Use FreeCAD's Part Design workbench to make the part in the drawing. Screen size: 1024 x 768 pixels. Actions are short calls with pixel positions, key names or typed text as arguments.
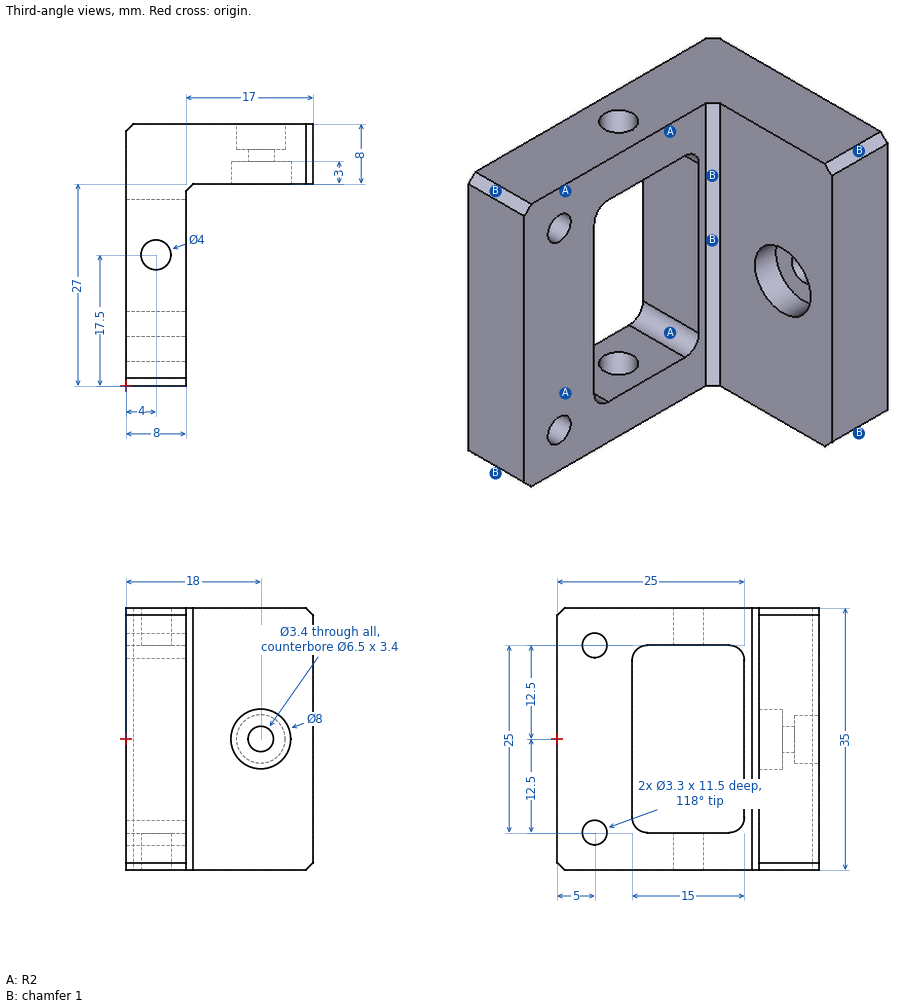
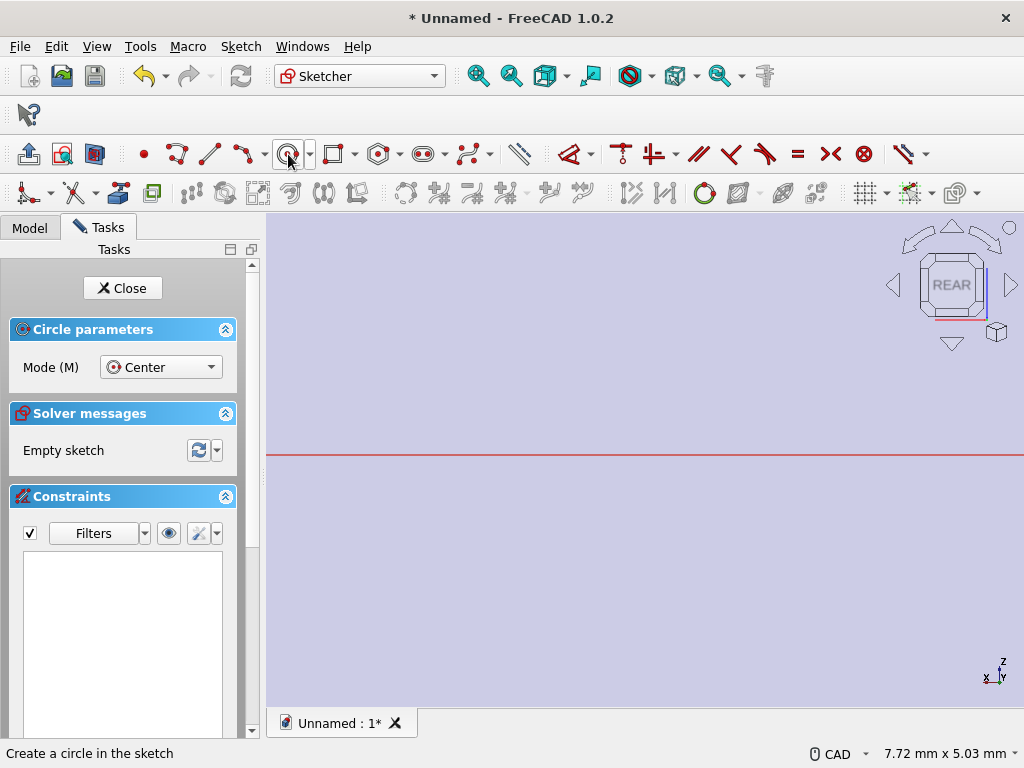
click(572, 455)
move(690, 337)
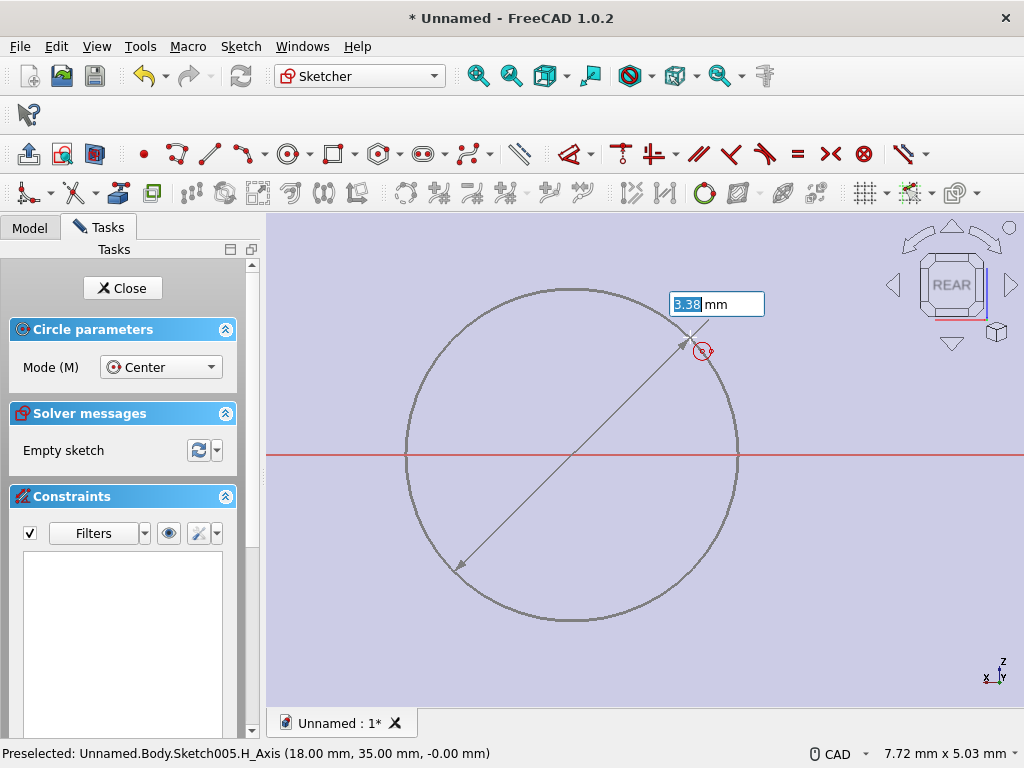
text(3.4)
key(Return)
key(Escape)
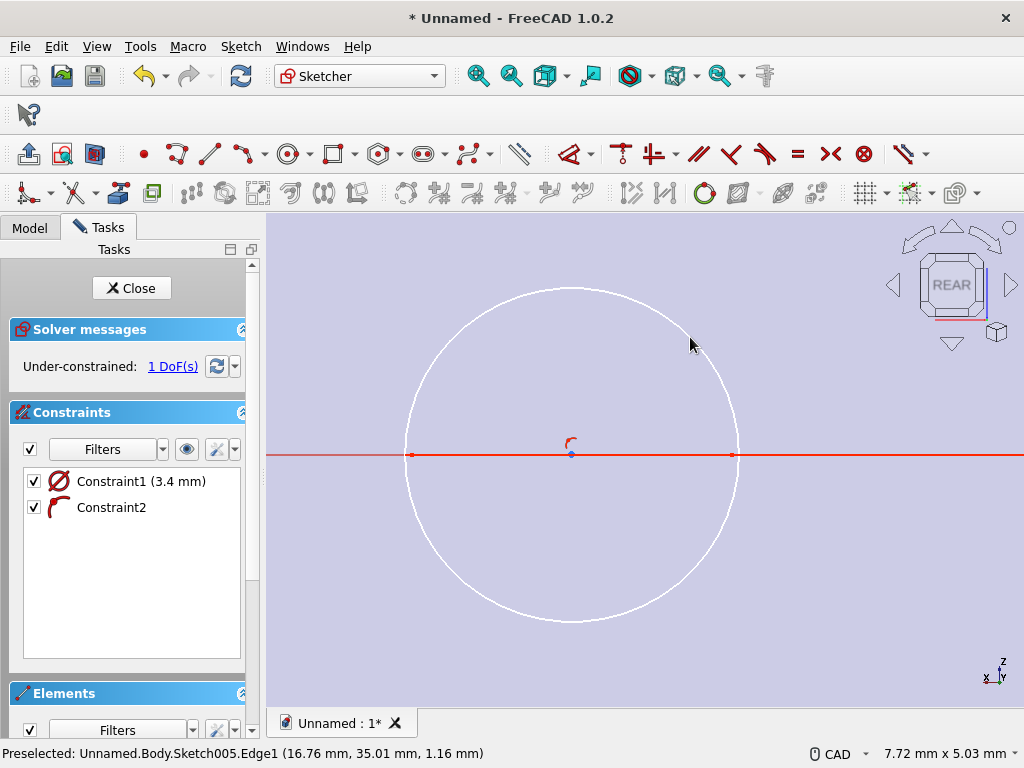
key(d)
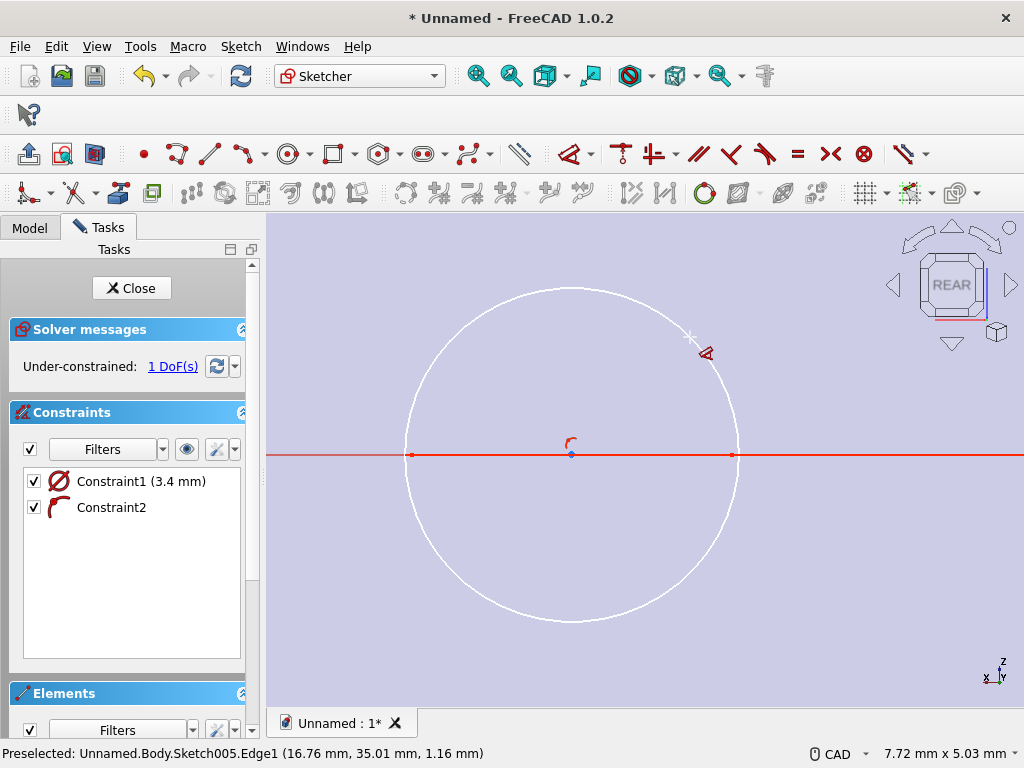
click(572, 455)
click(716, 489)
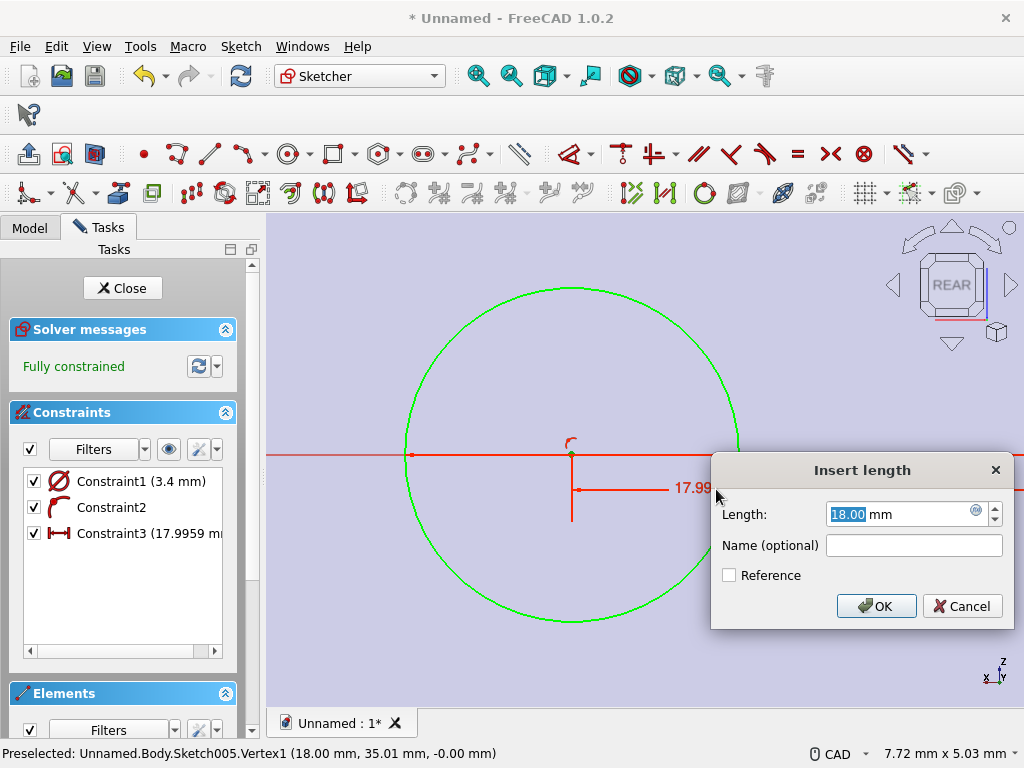
text(18)
key(Return)
key(Escape)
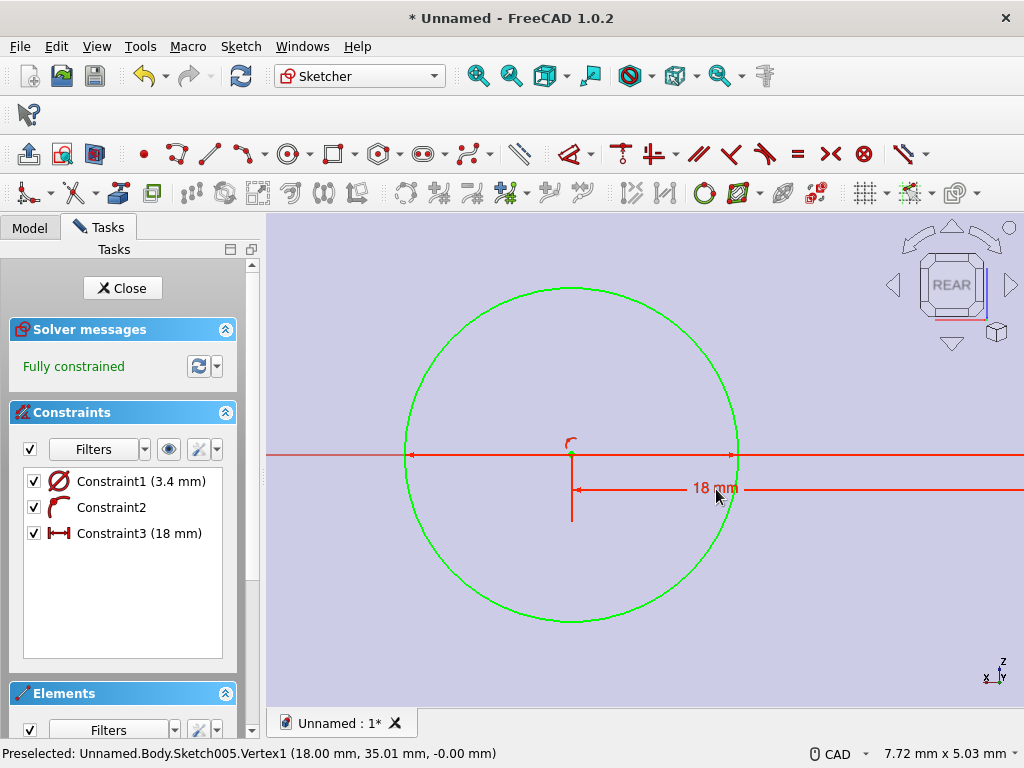
click(123, 288)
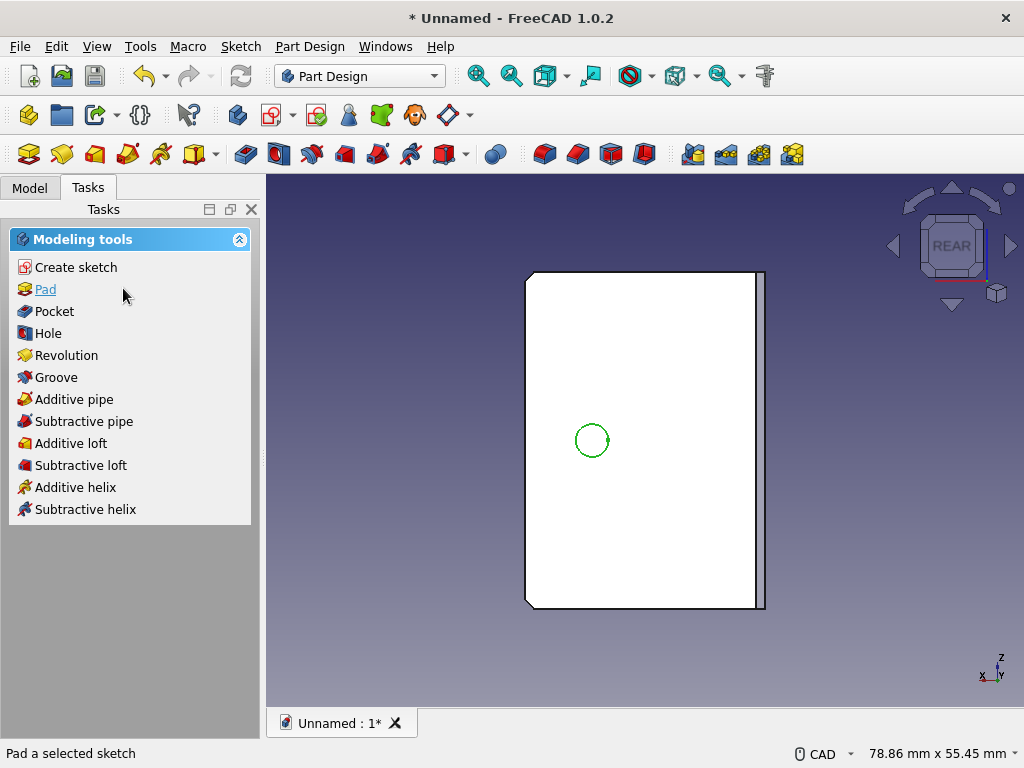
click(279, 154)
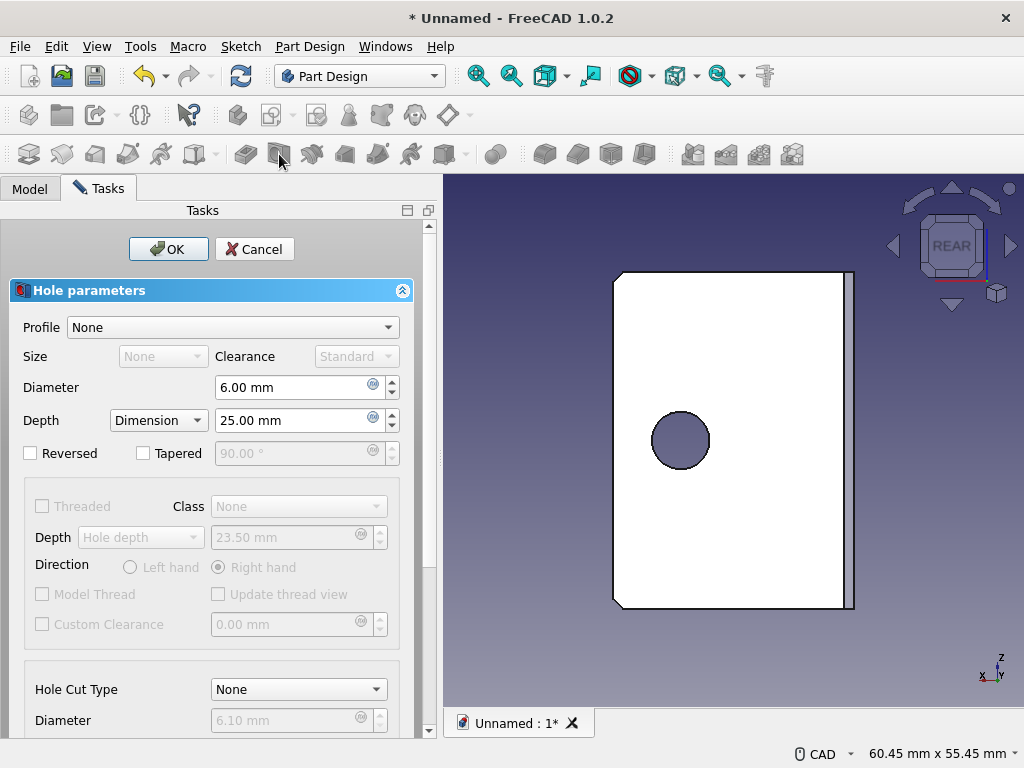
triple_click(300, 388)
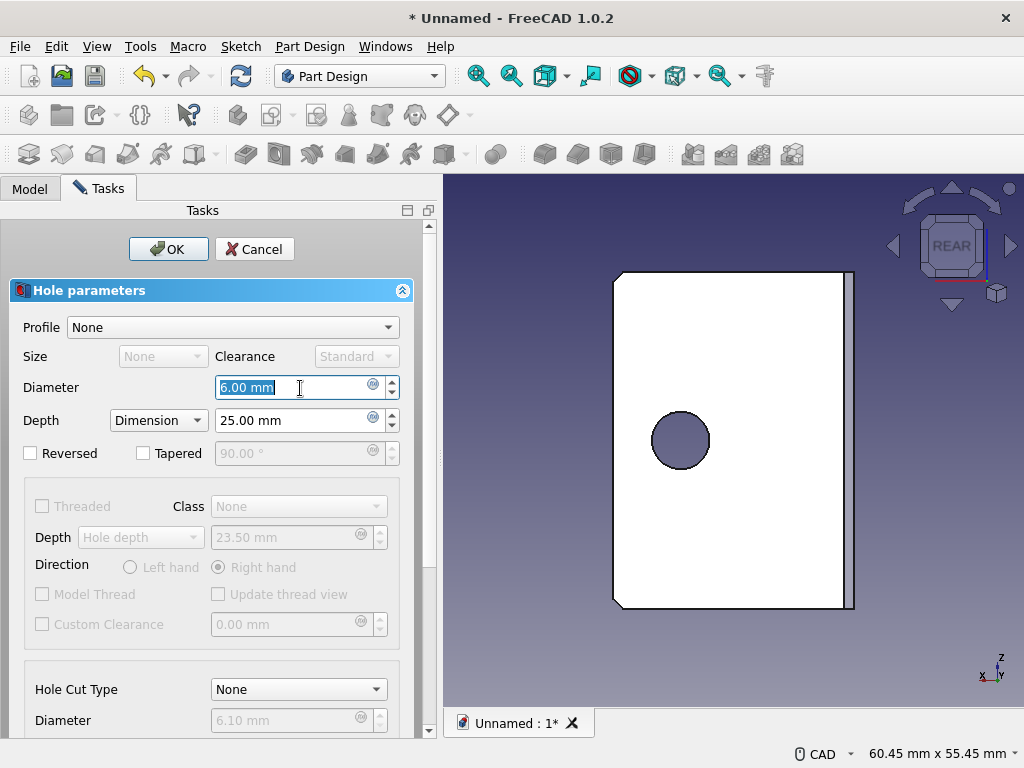
text(3.4)
key(Tab)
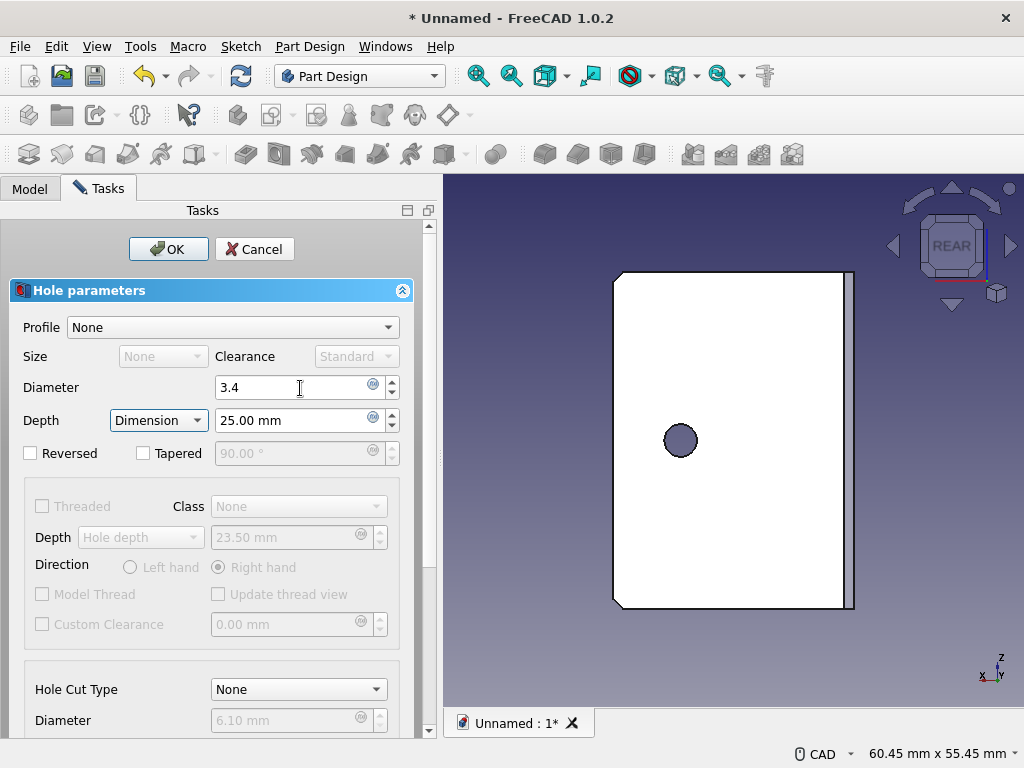
click(160, 420)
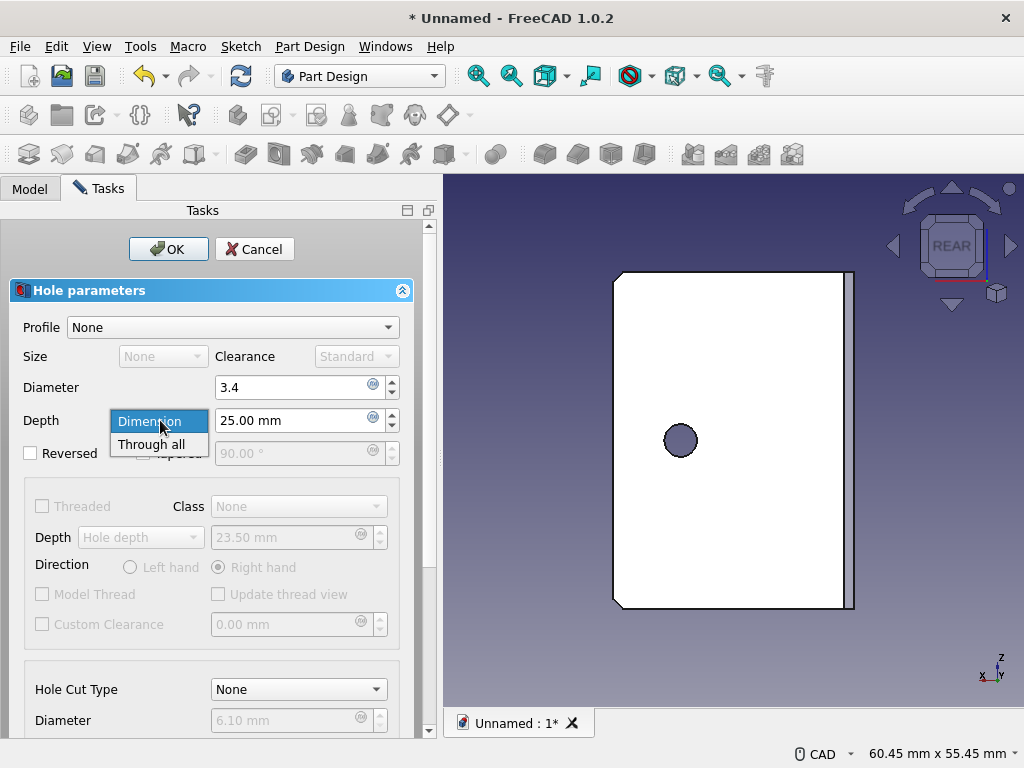
click(158, 444)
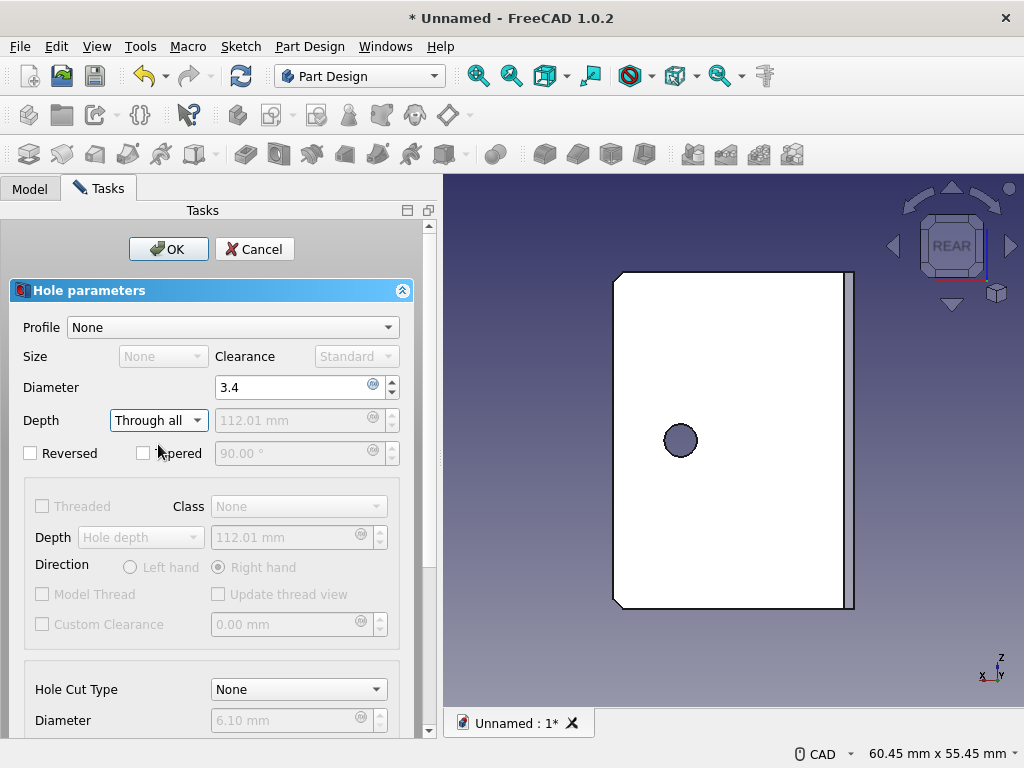
click(300, 690)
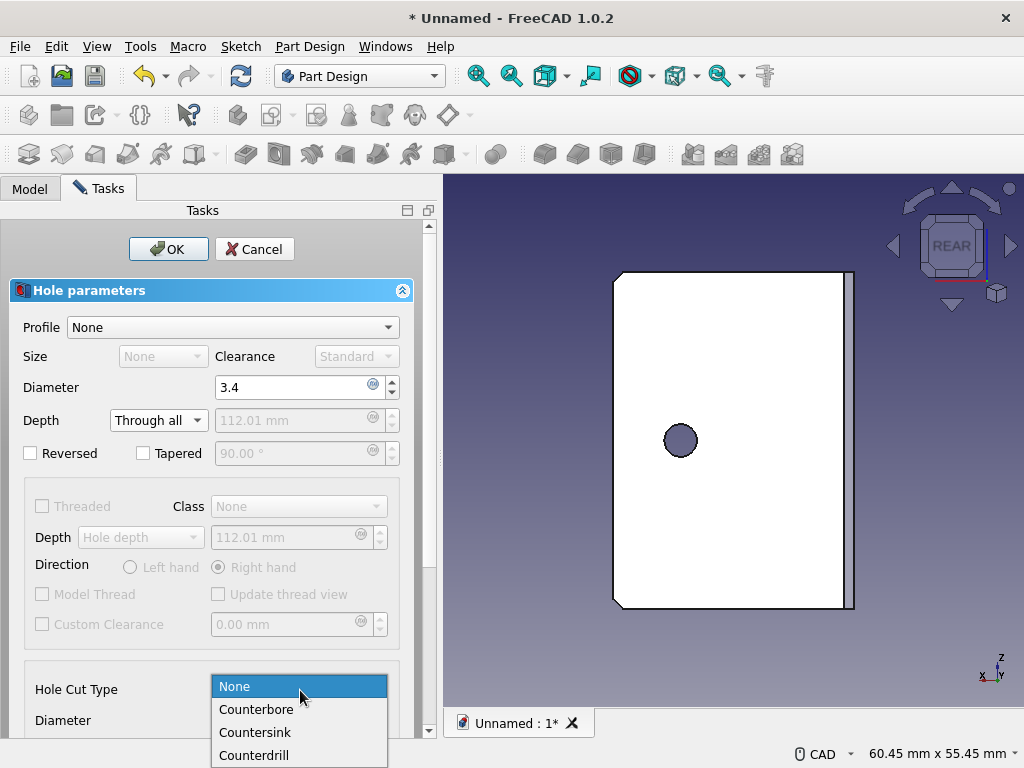
click(298, 710)